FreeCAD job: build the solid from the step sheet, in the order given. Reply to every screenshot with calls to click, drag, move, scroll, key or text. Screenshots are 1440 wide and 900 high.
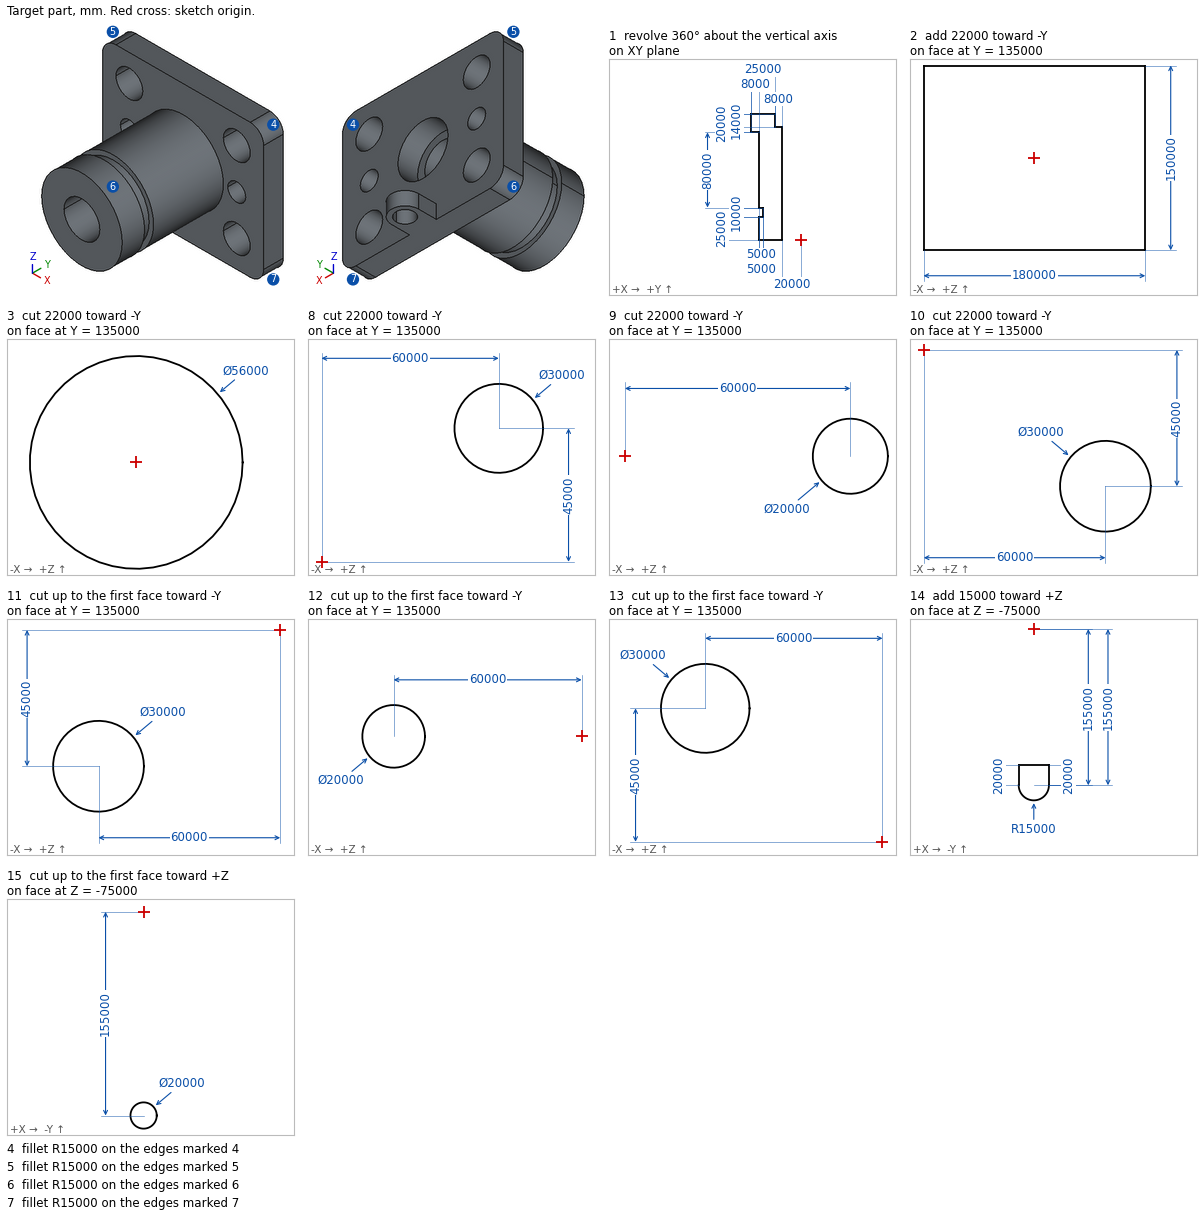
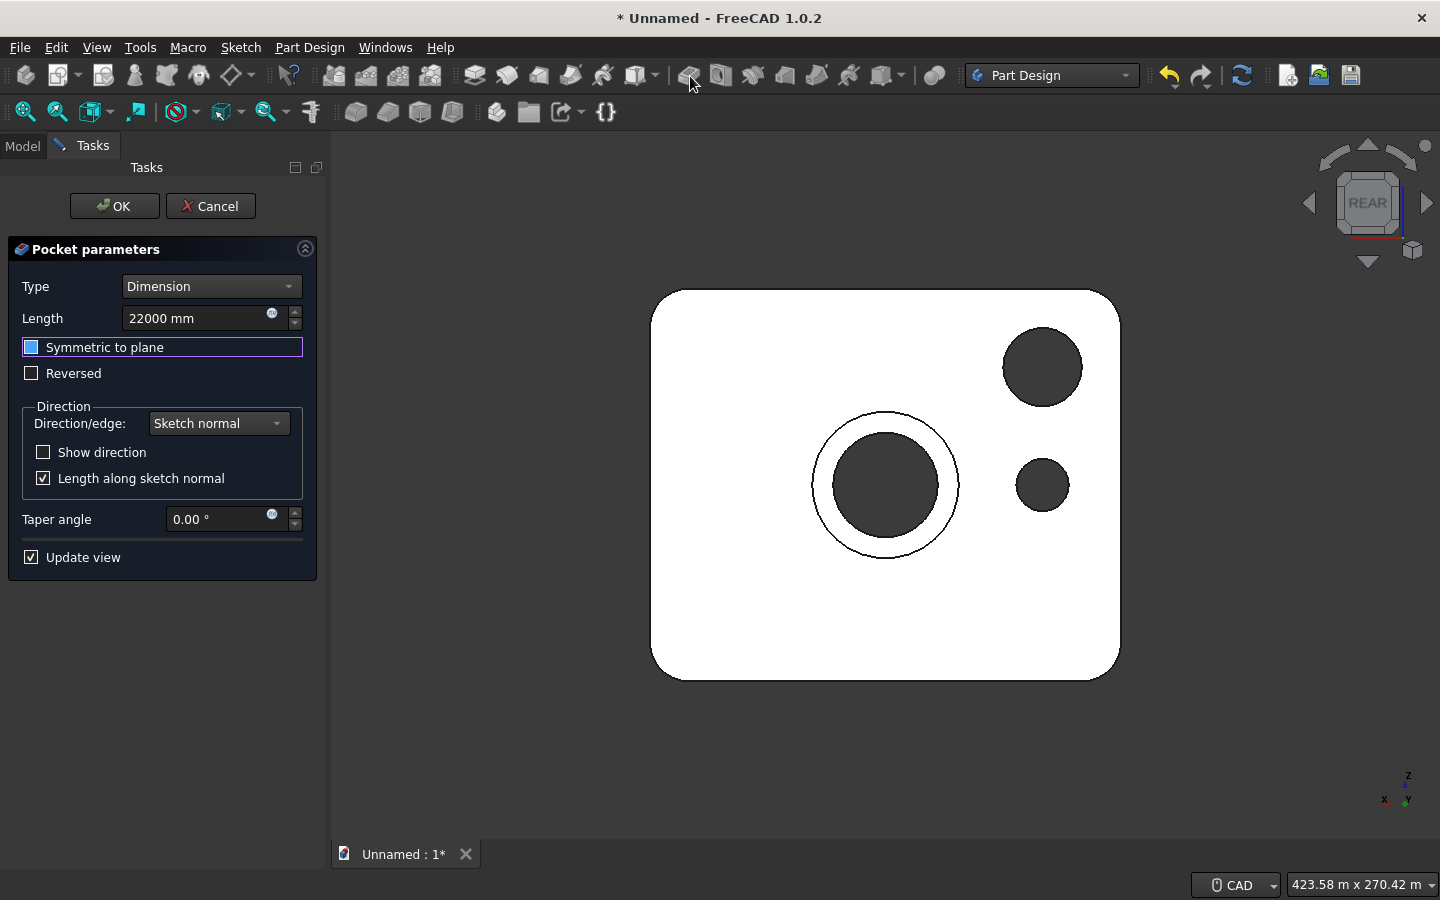
click(115, 206)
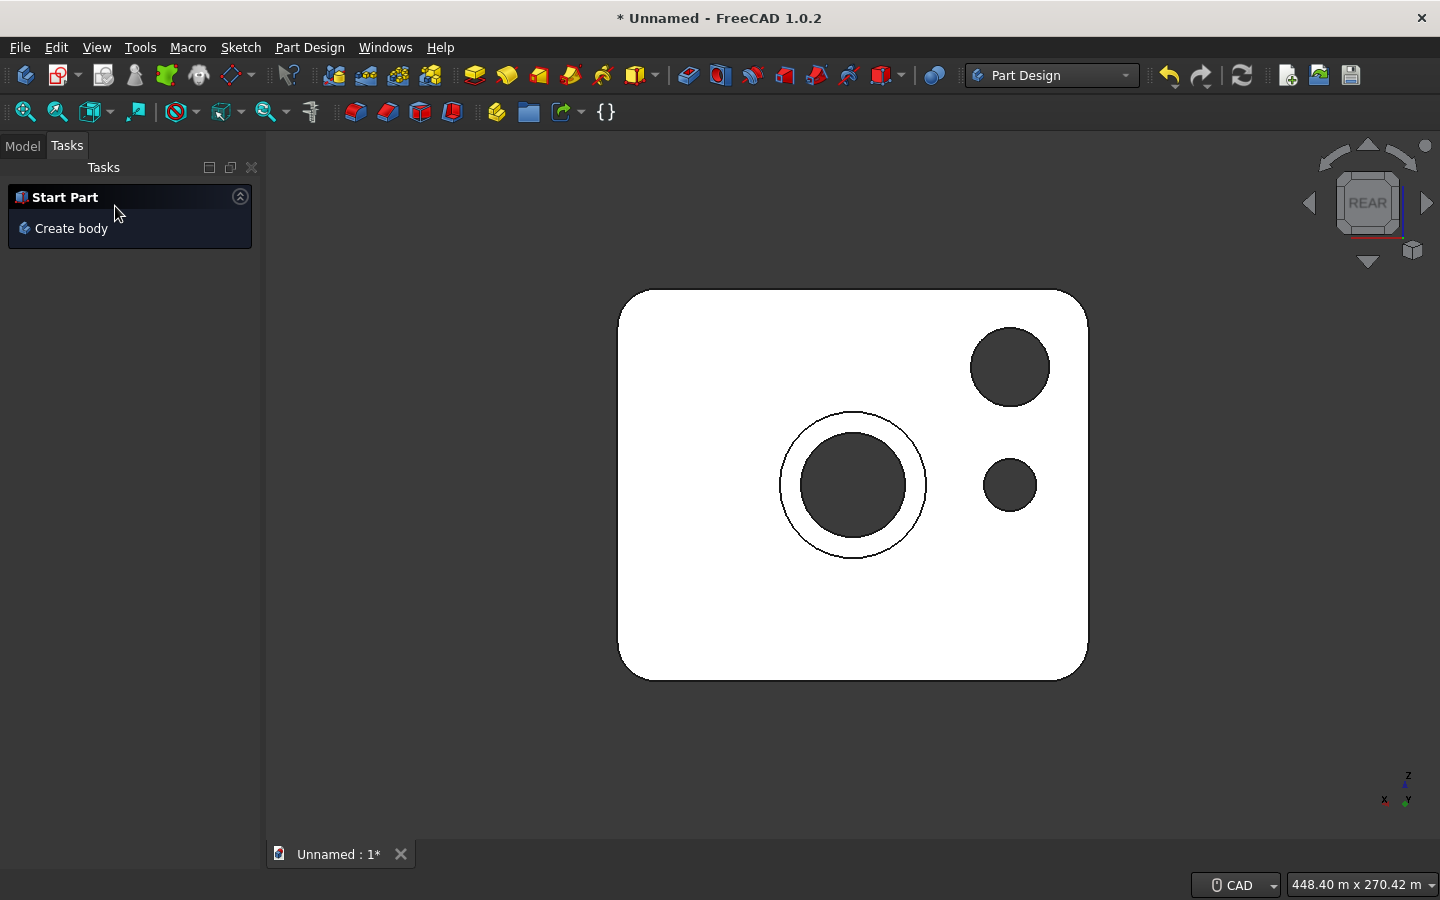
click(718, 372)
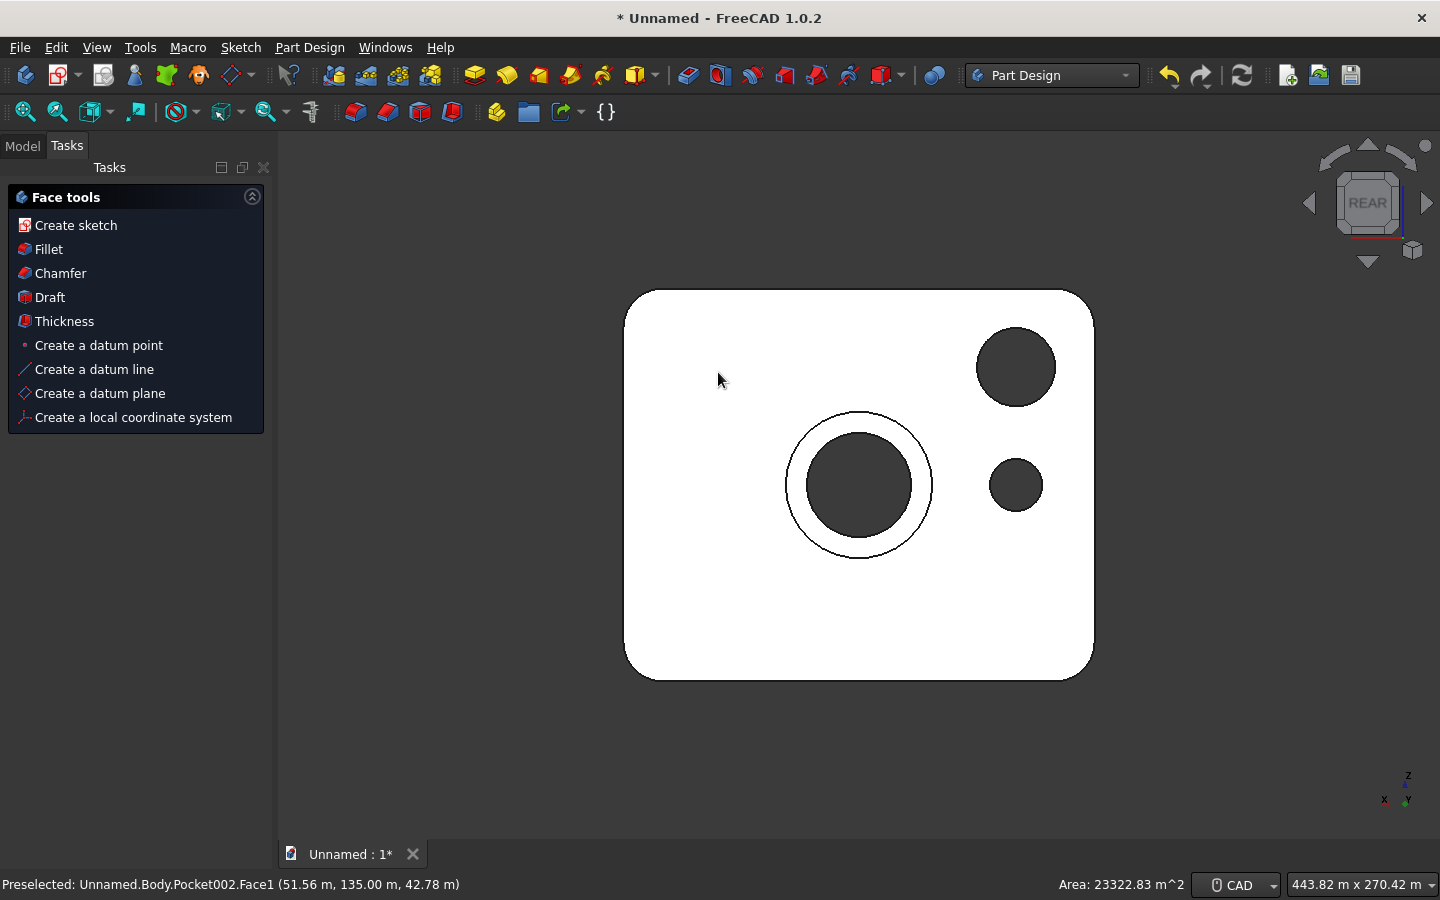
click(58, 76)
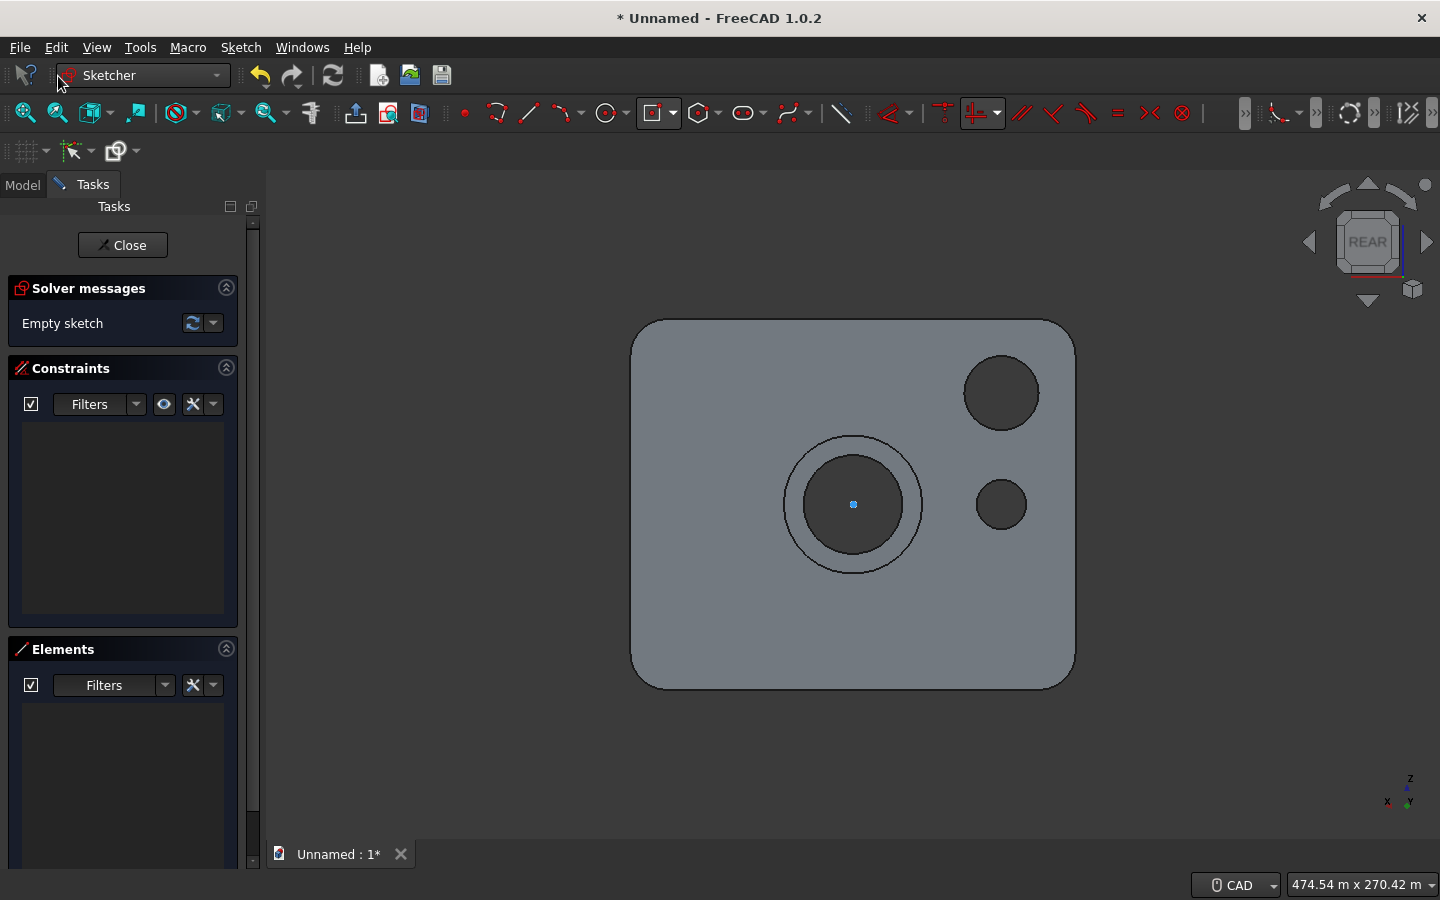
scroll(1044, 638, up, 9)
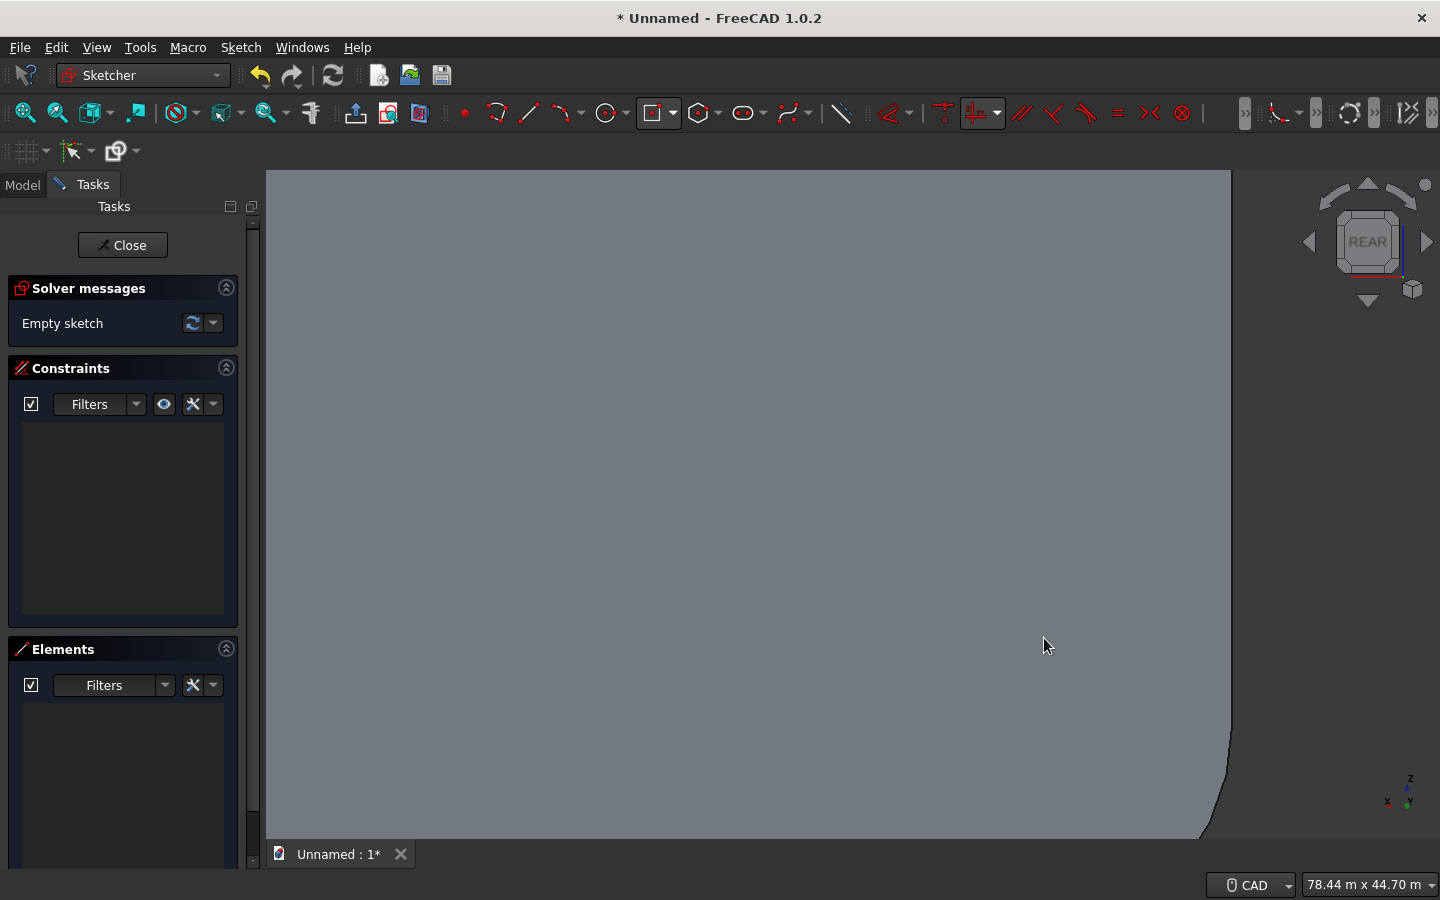
click(606, 114)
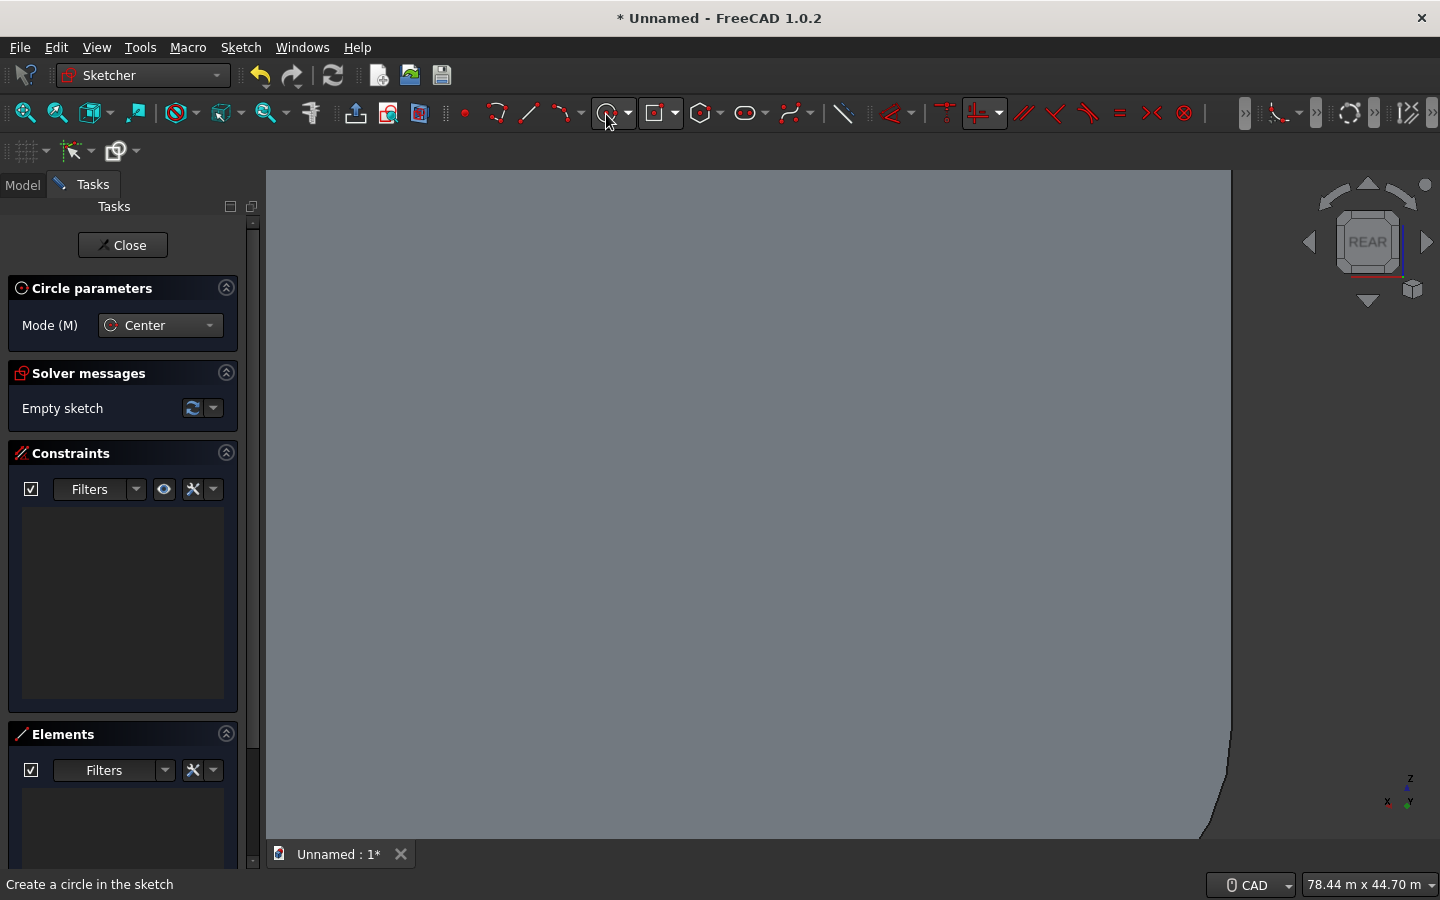
click(783, 500)
click(942, 342)
key(Escape)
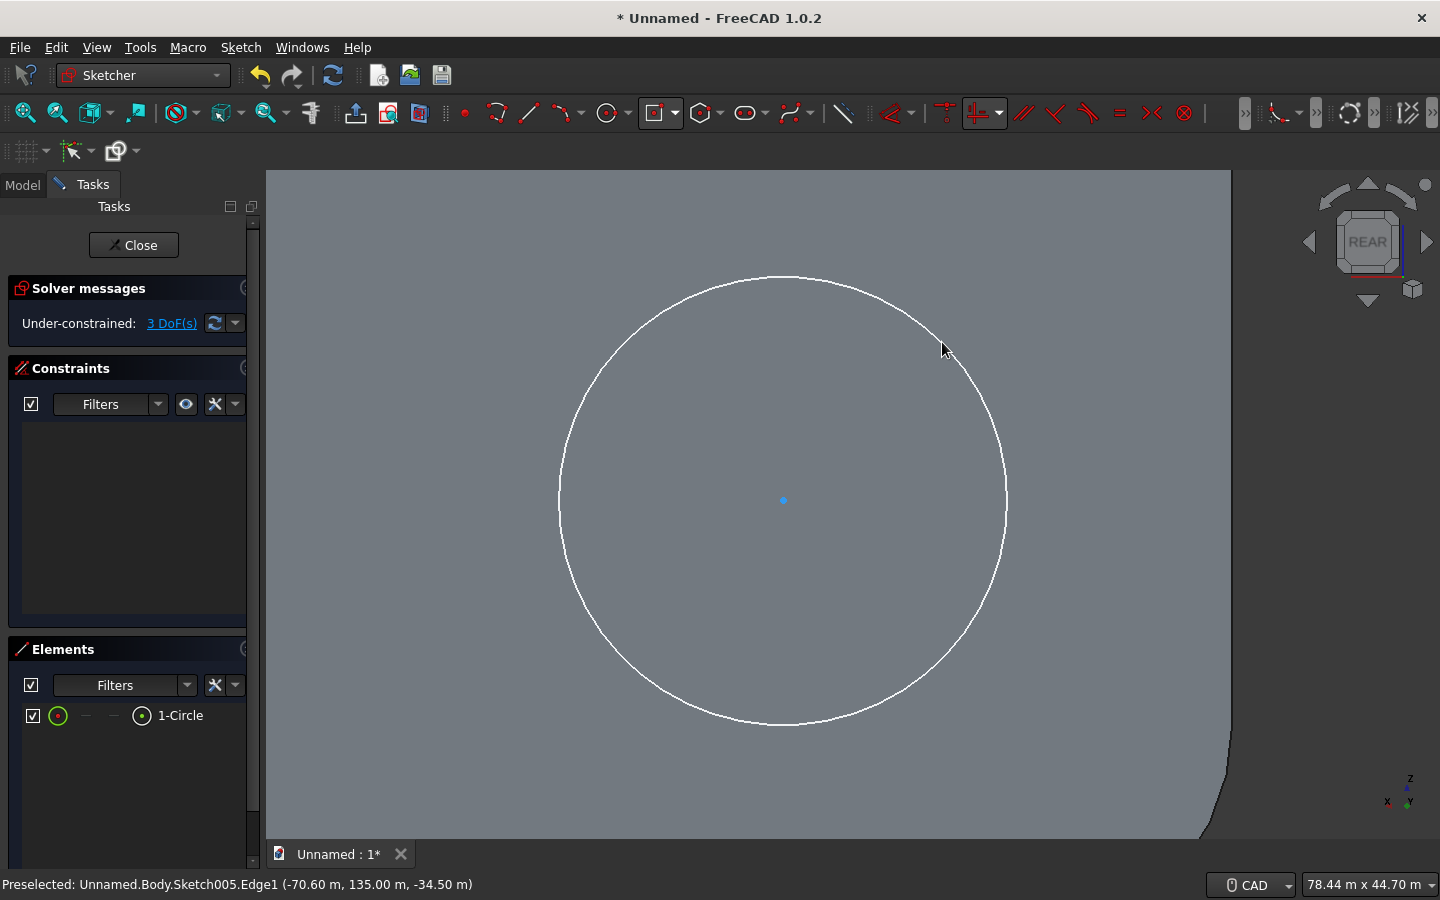
key(d)